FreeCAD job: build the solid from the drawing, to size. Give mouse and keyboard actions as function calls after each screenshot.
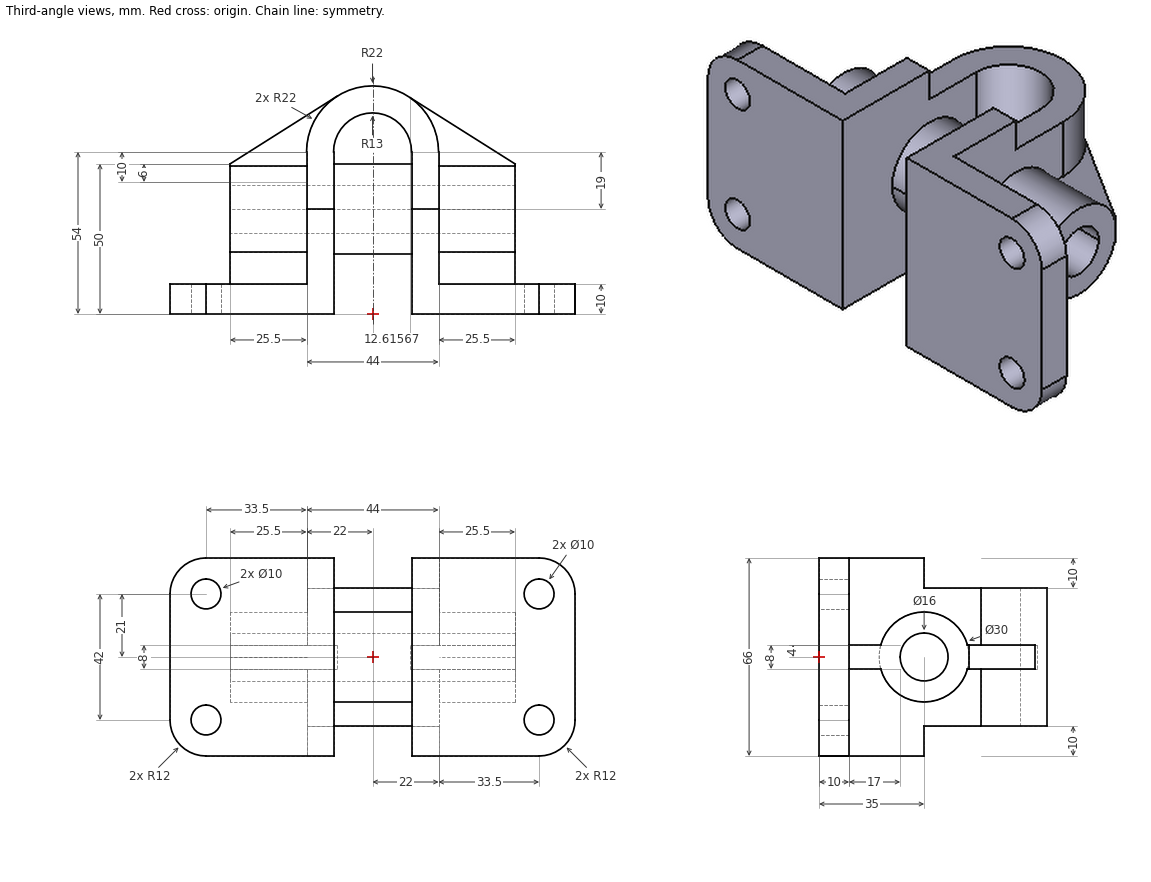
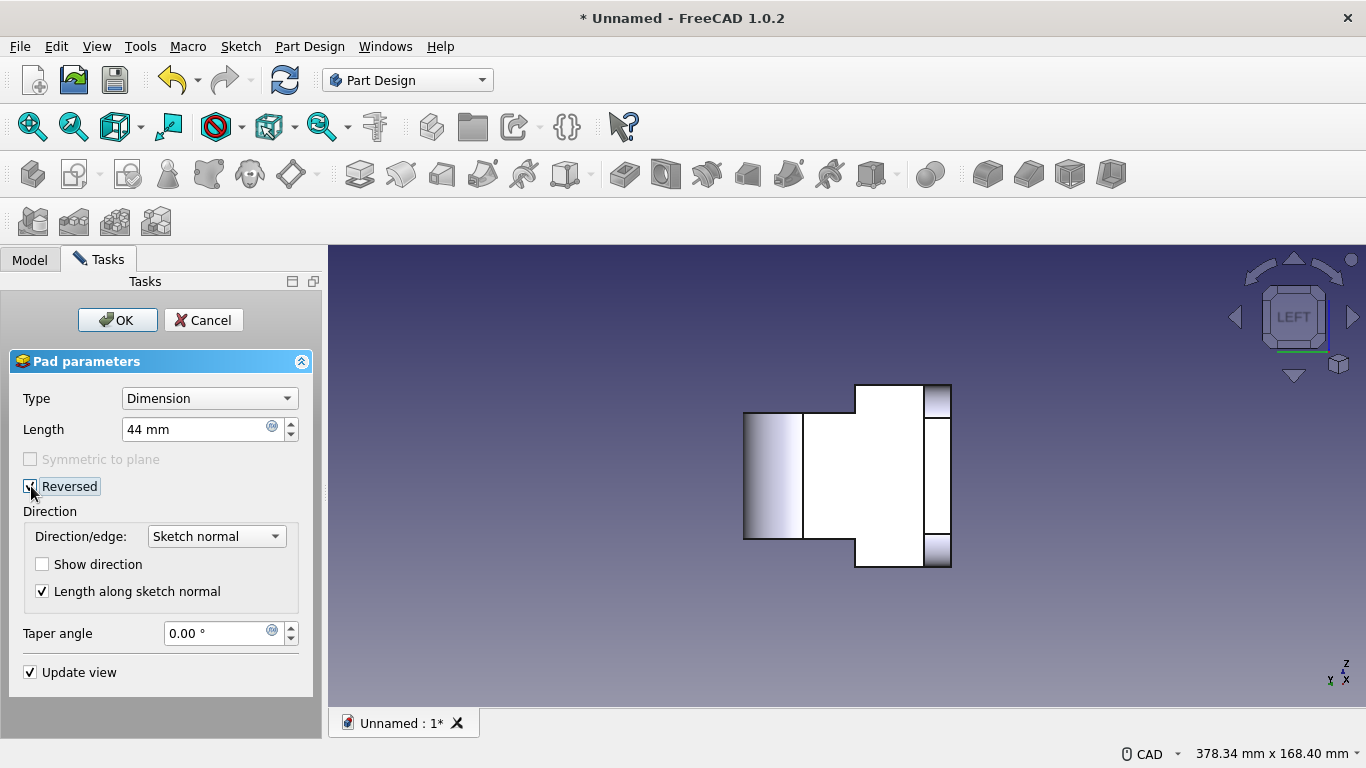
click(118, 320)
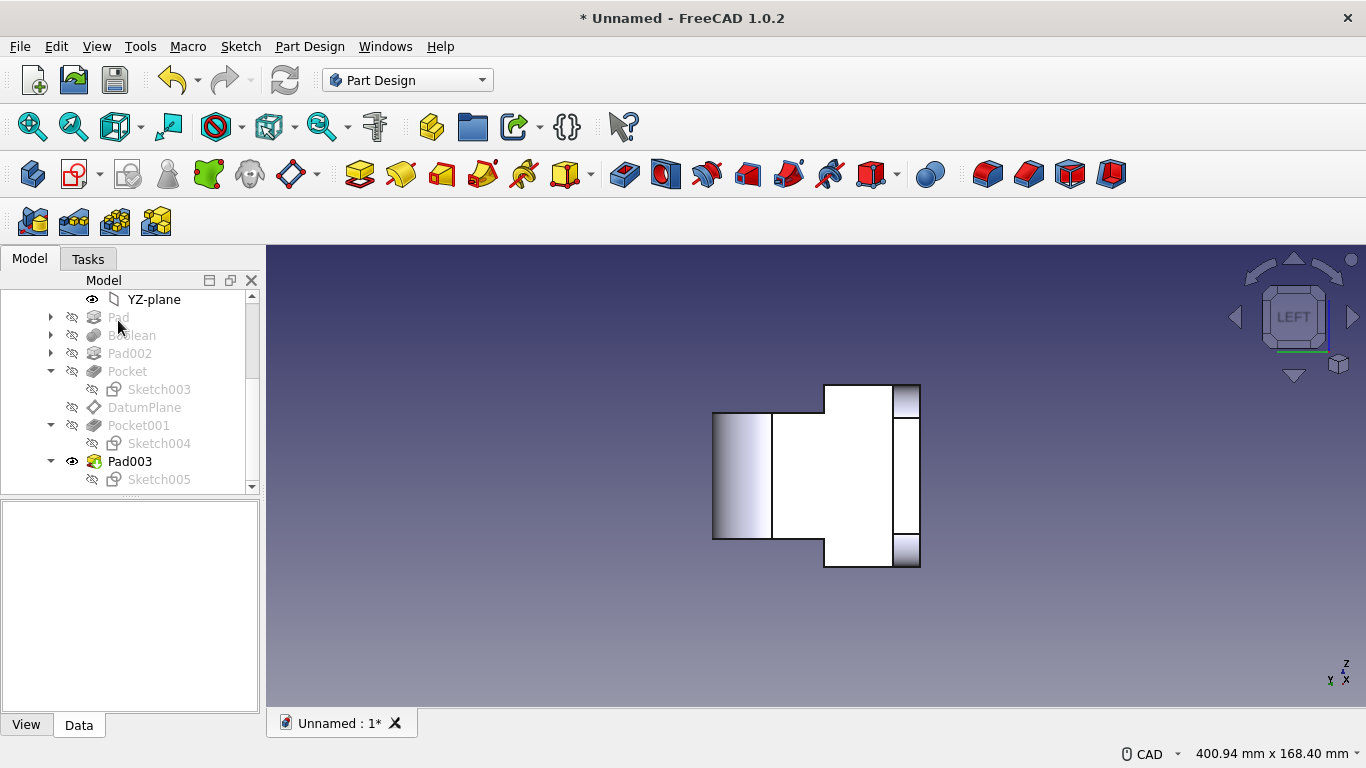
click(33, 128)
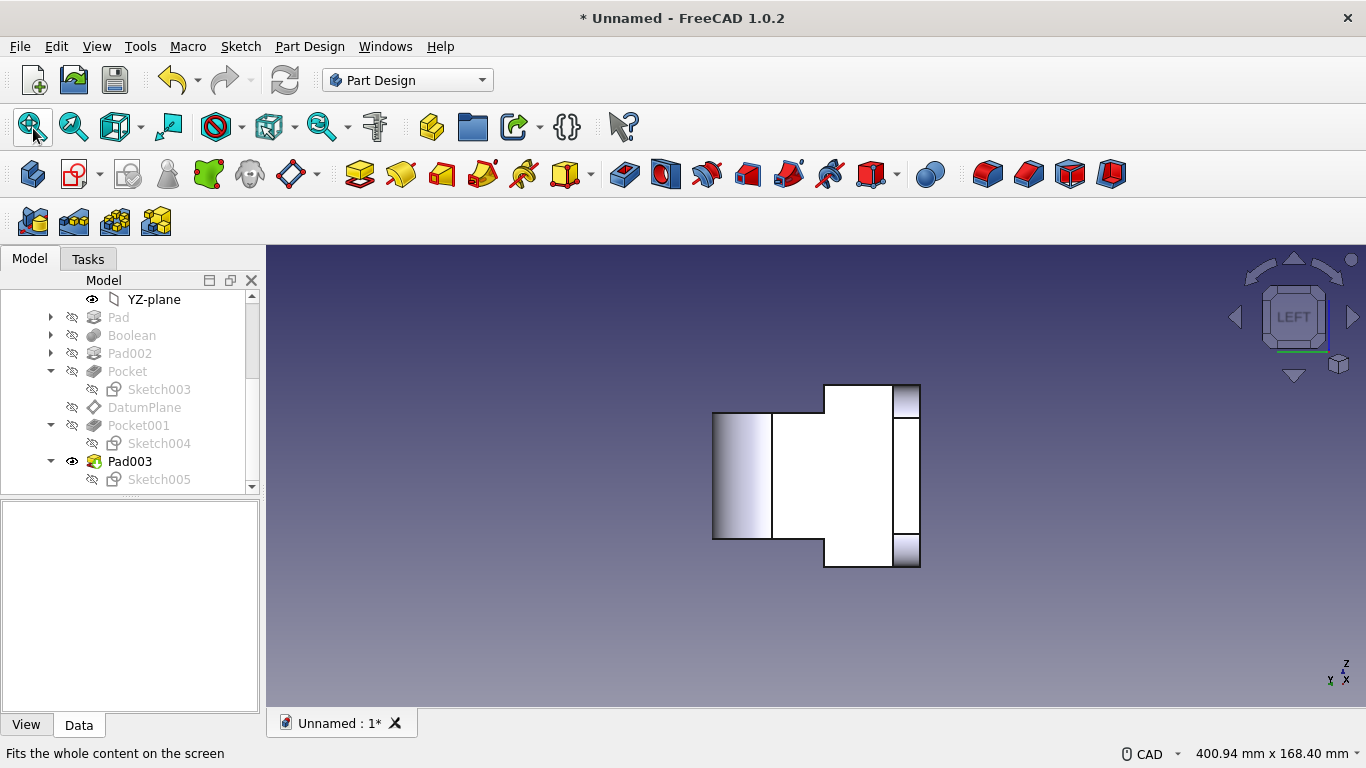
click(832, 475)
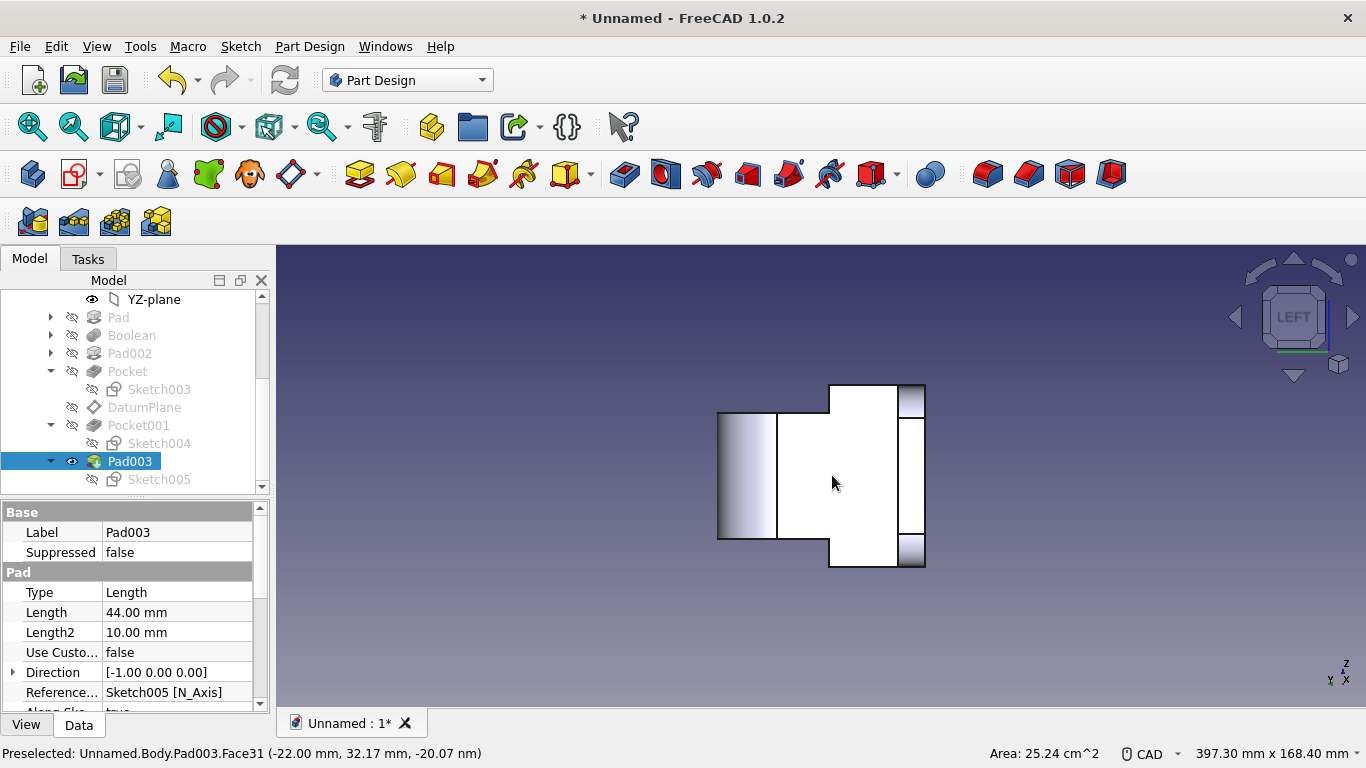
click(74, 174)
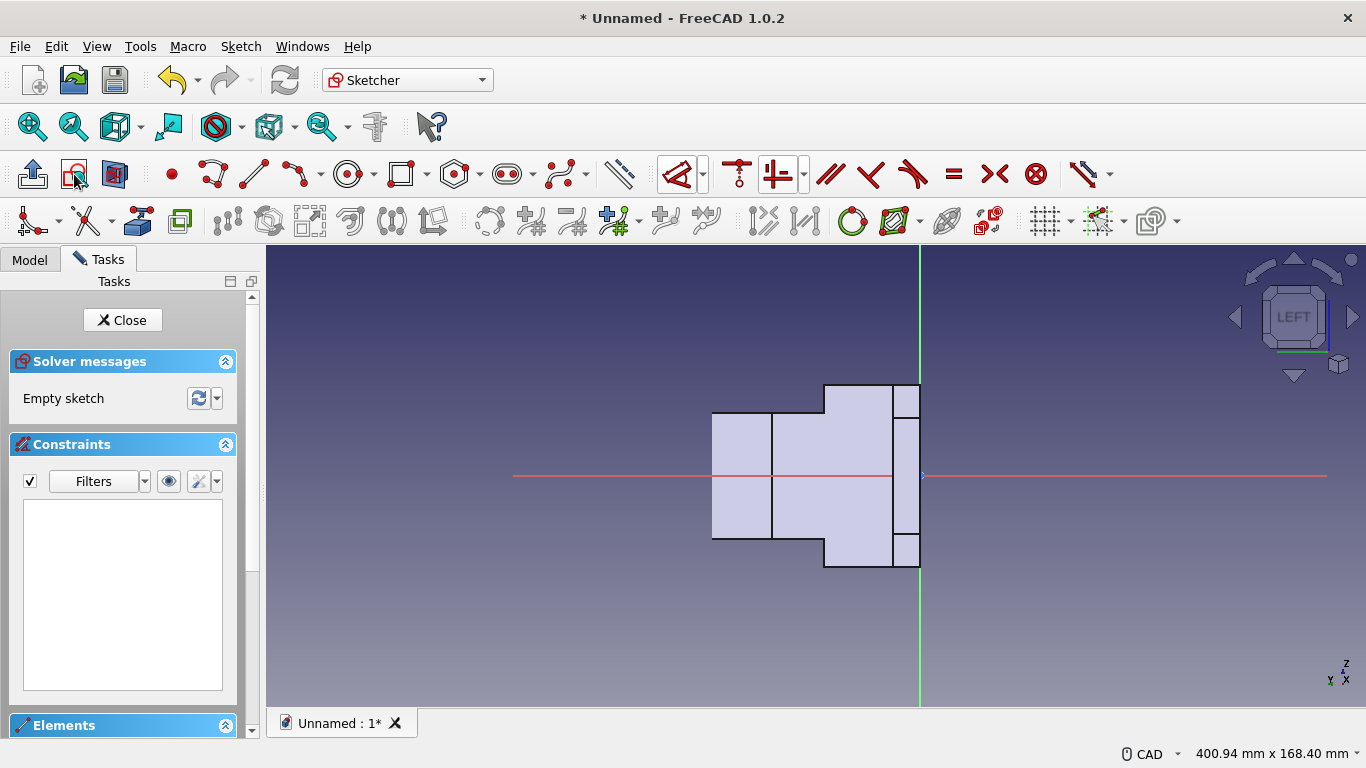
scroll(839, 476, up, 9)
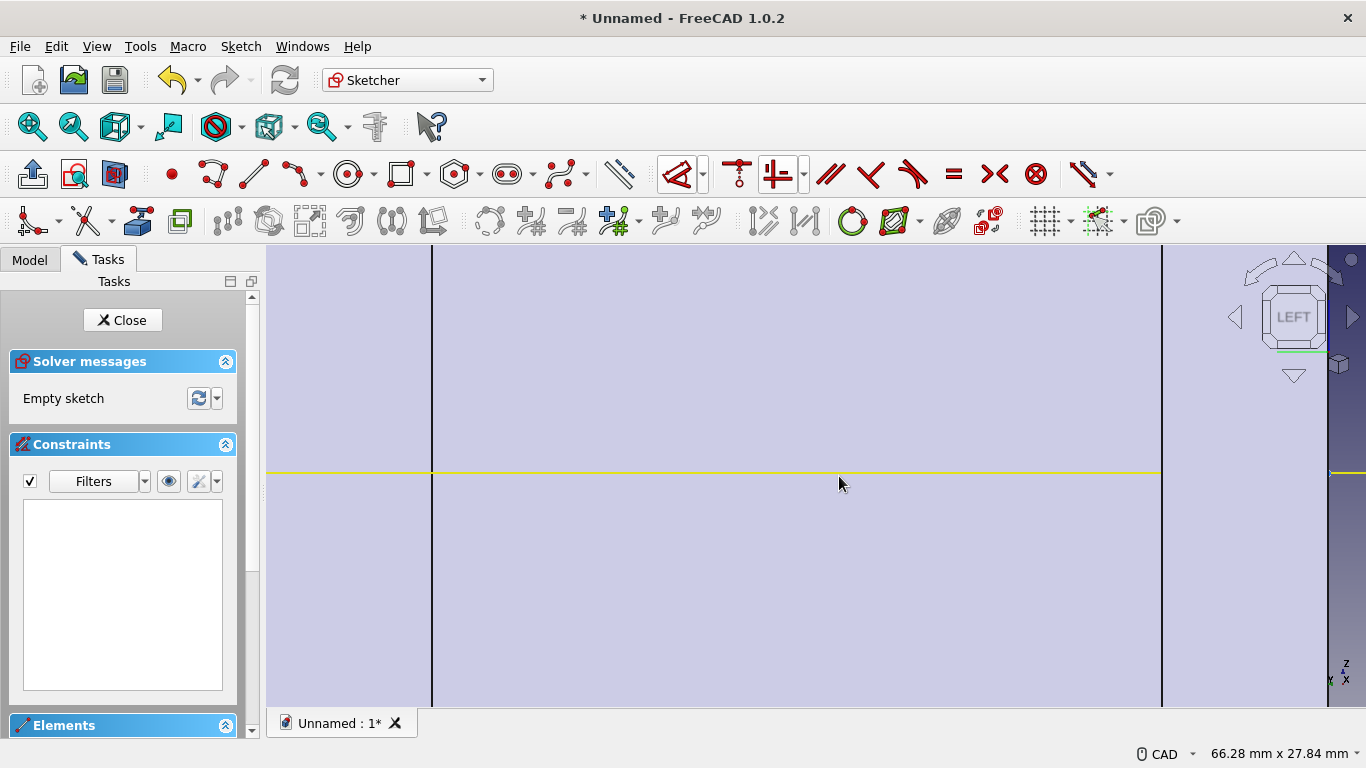
click(348, 174)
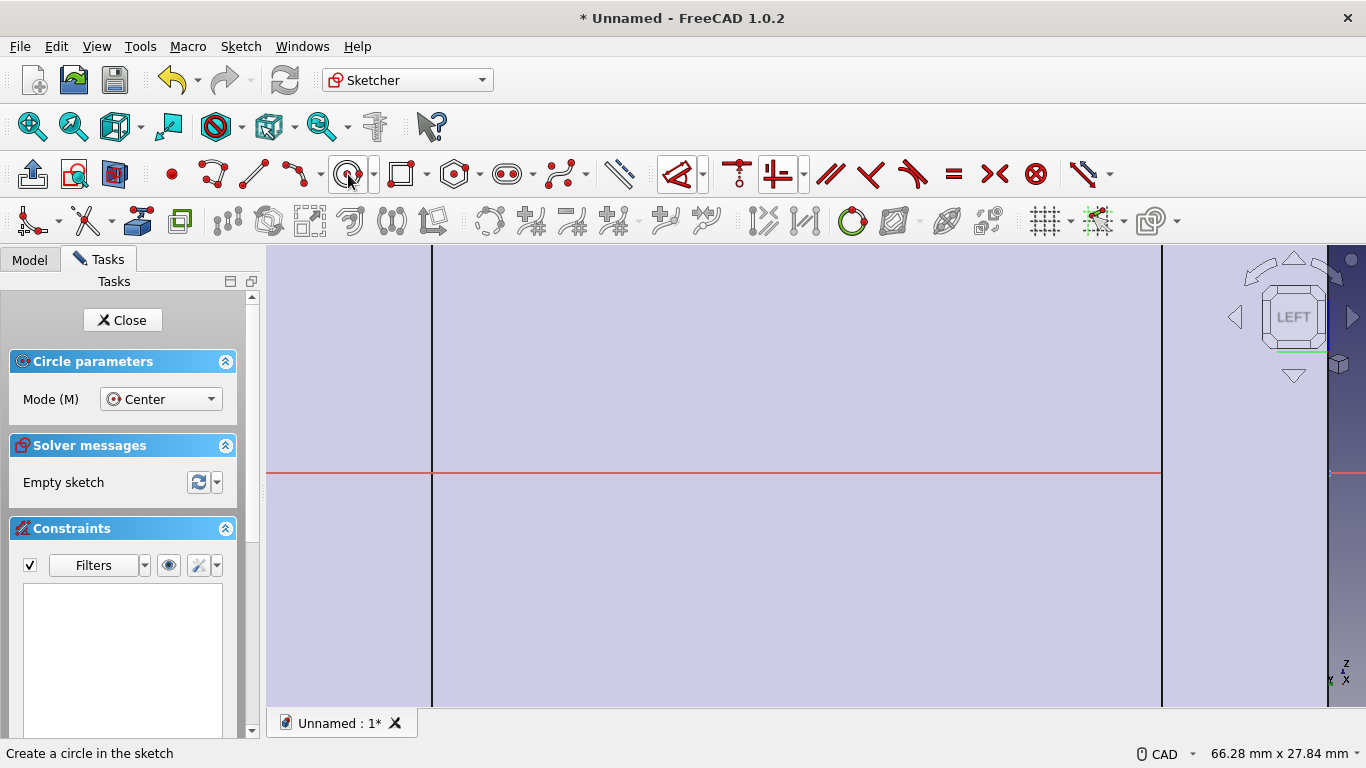
click(747, 473)
move(841, 380)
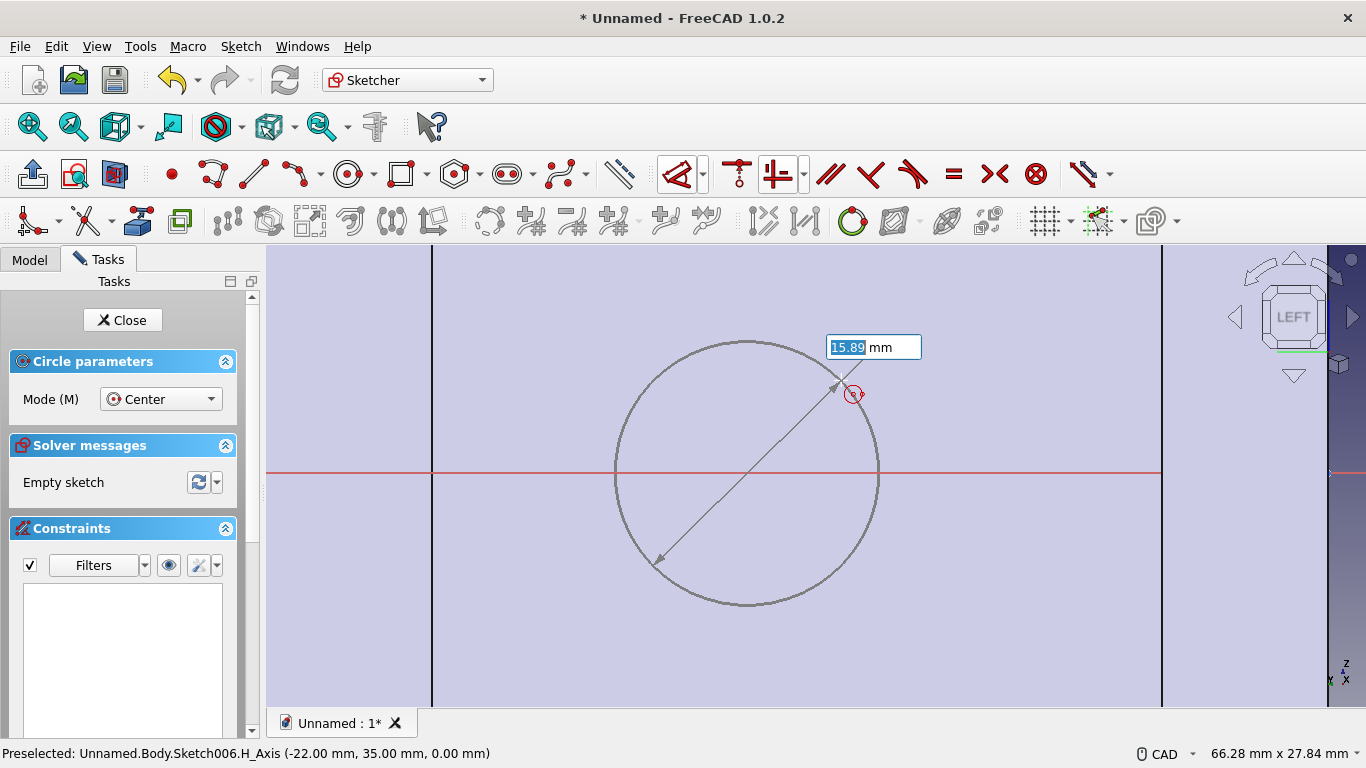
text(16)
key(Return)
key(Escape)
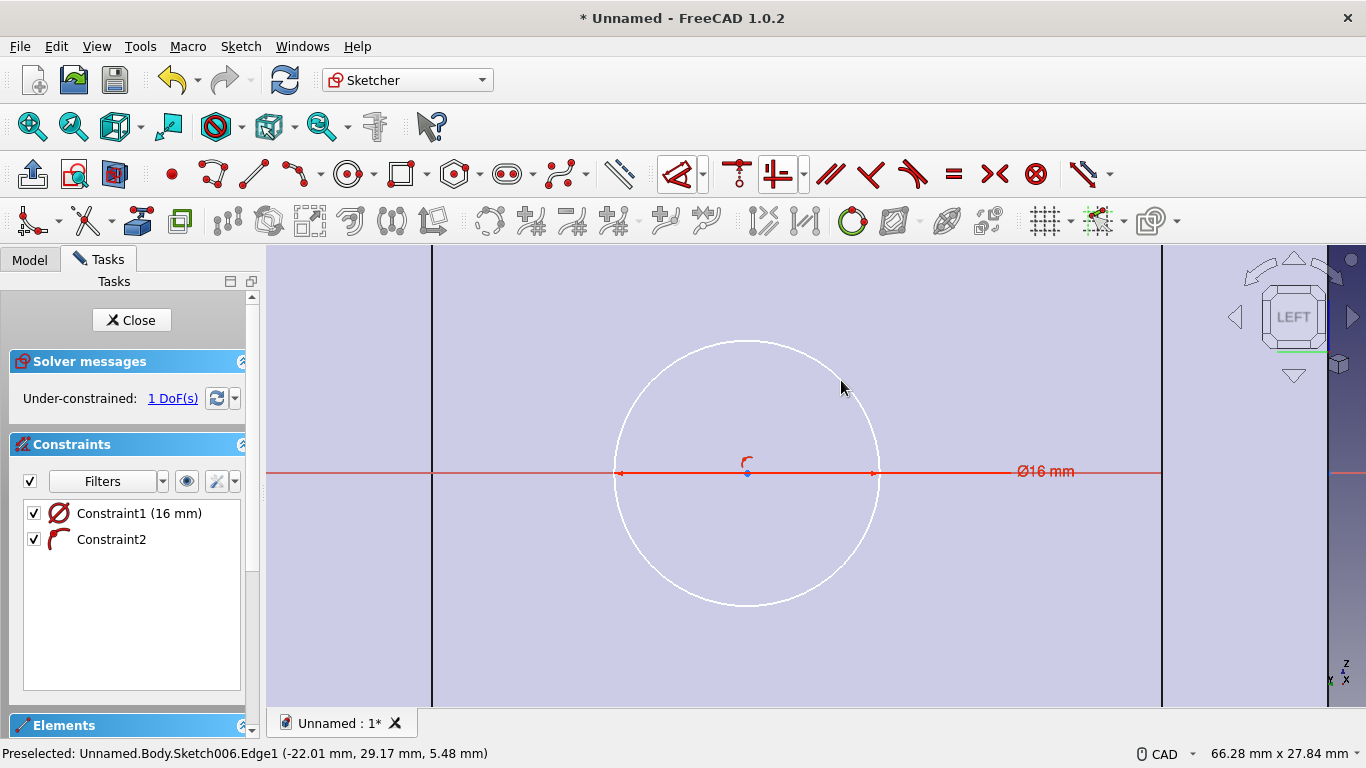
click(747, 473)